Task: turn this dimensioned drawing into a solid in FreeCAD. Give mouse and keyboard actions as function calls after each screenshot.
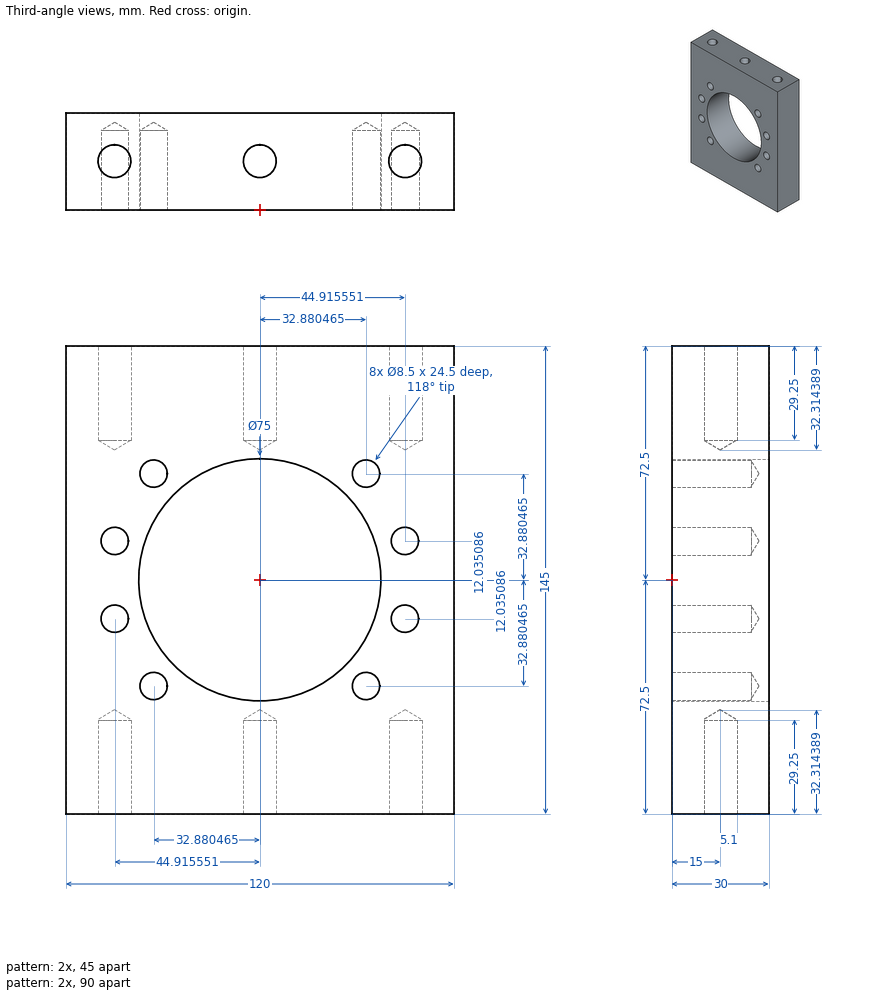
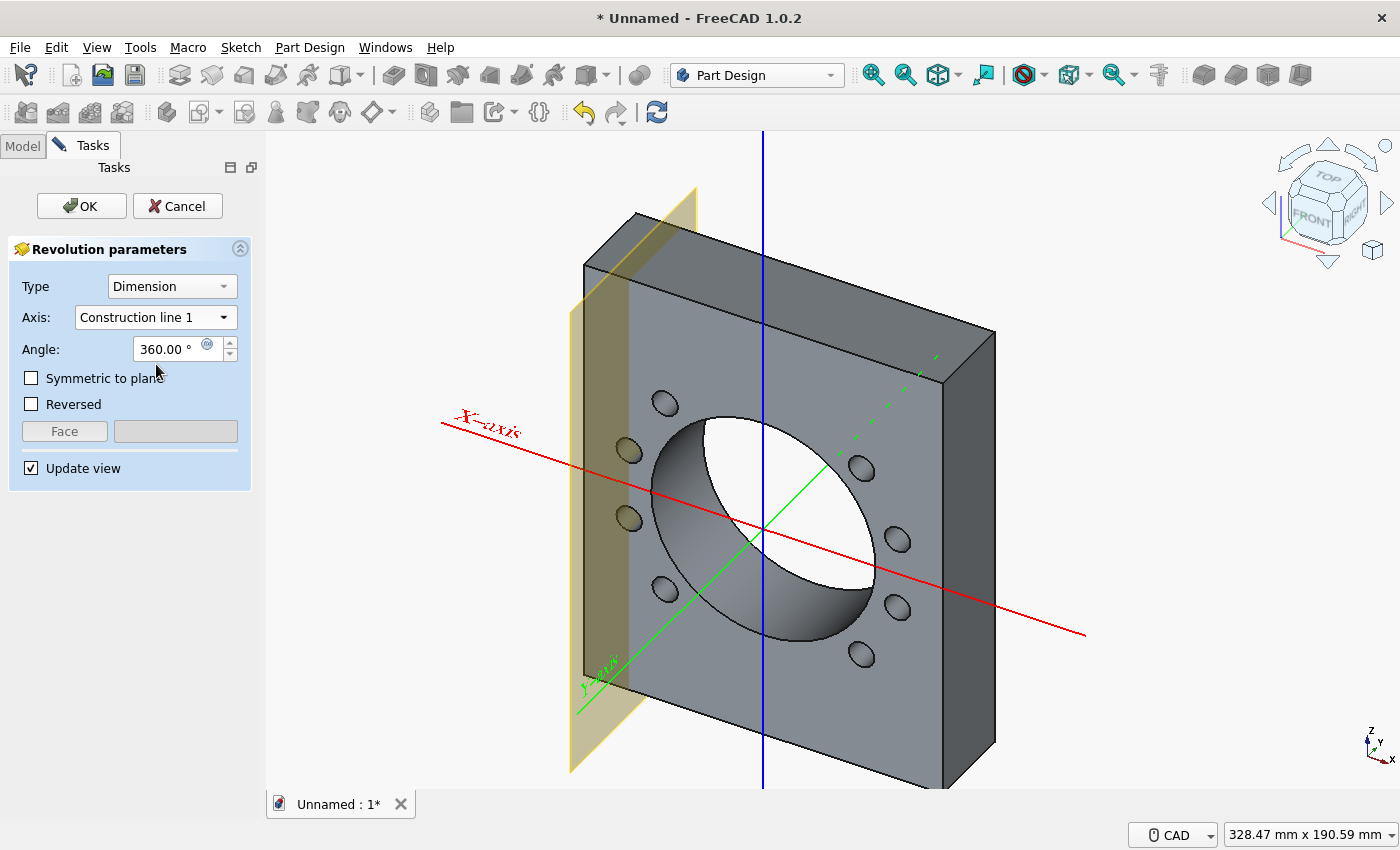
click(82, 206)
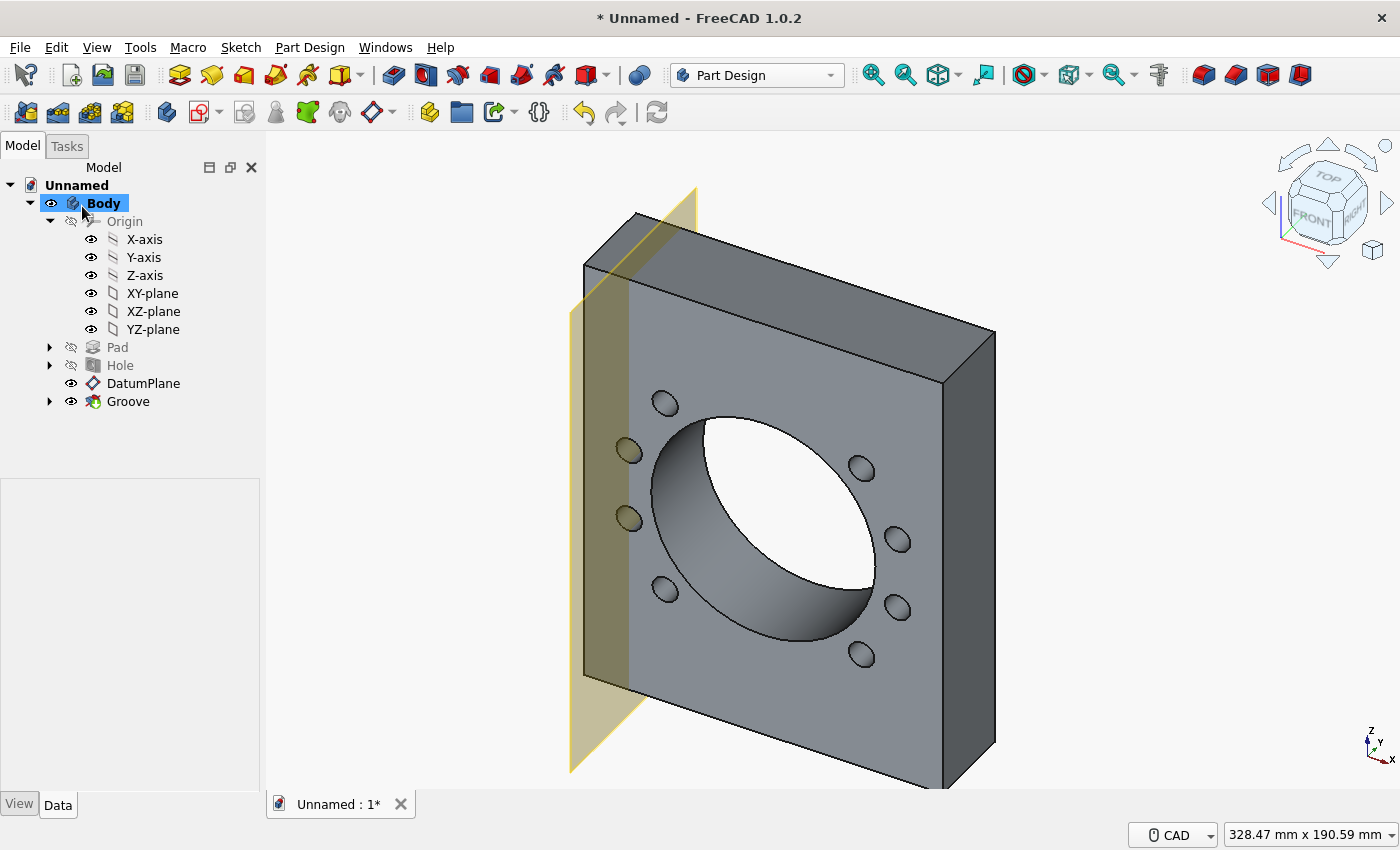
click(116, 383)
key(space)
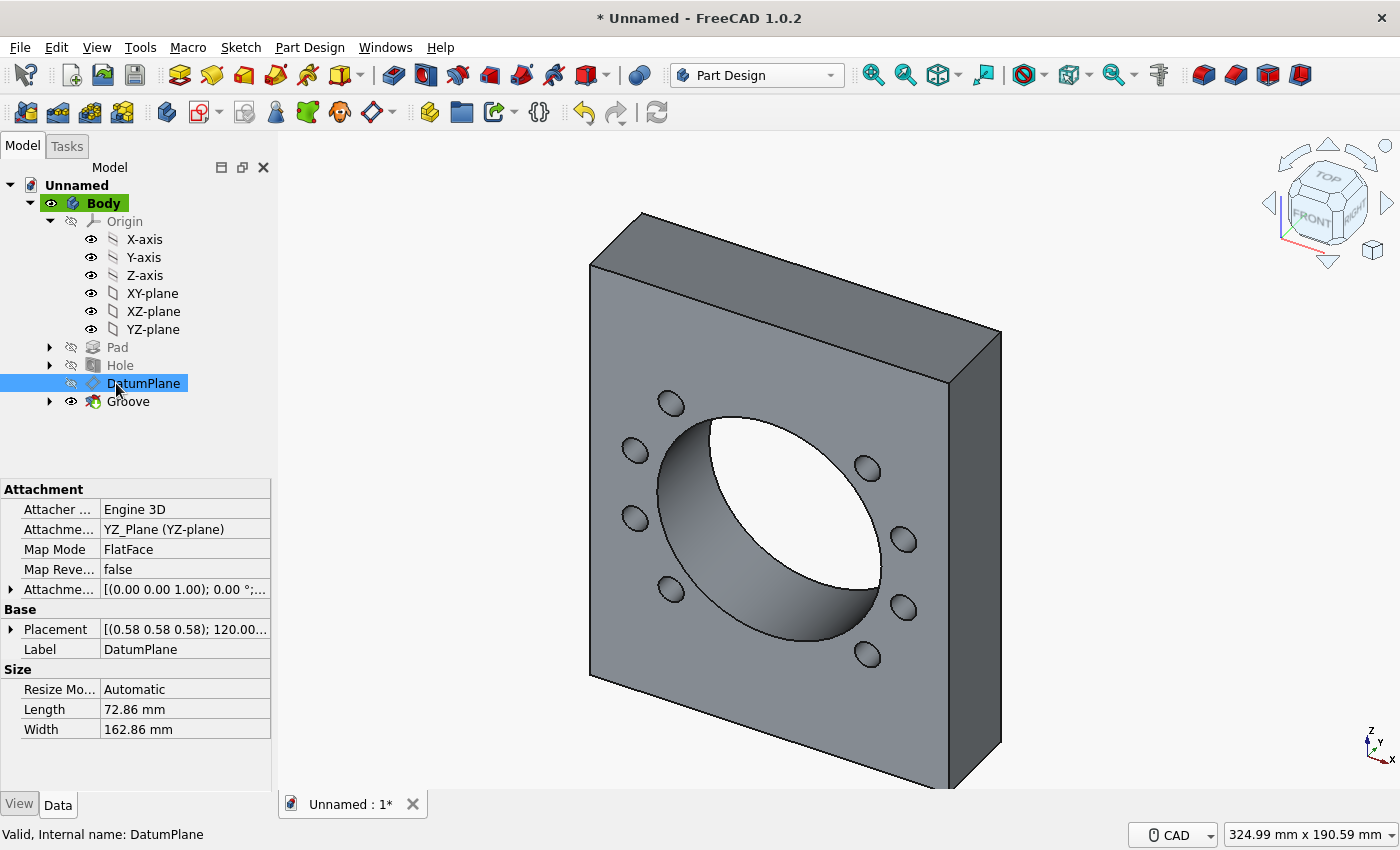
click(874, 76)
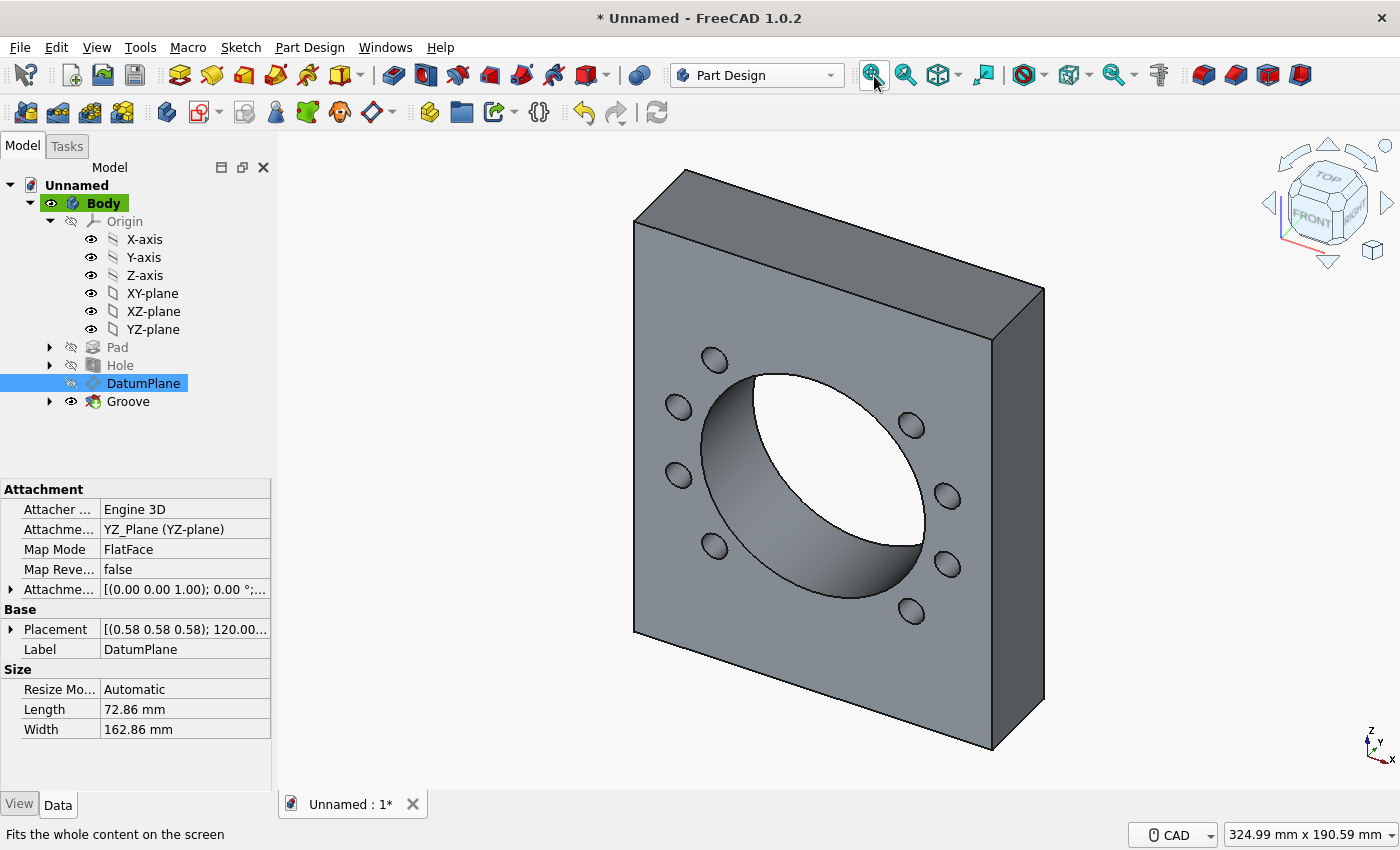
click(116, 401)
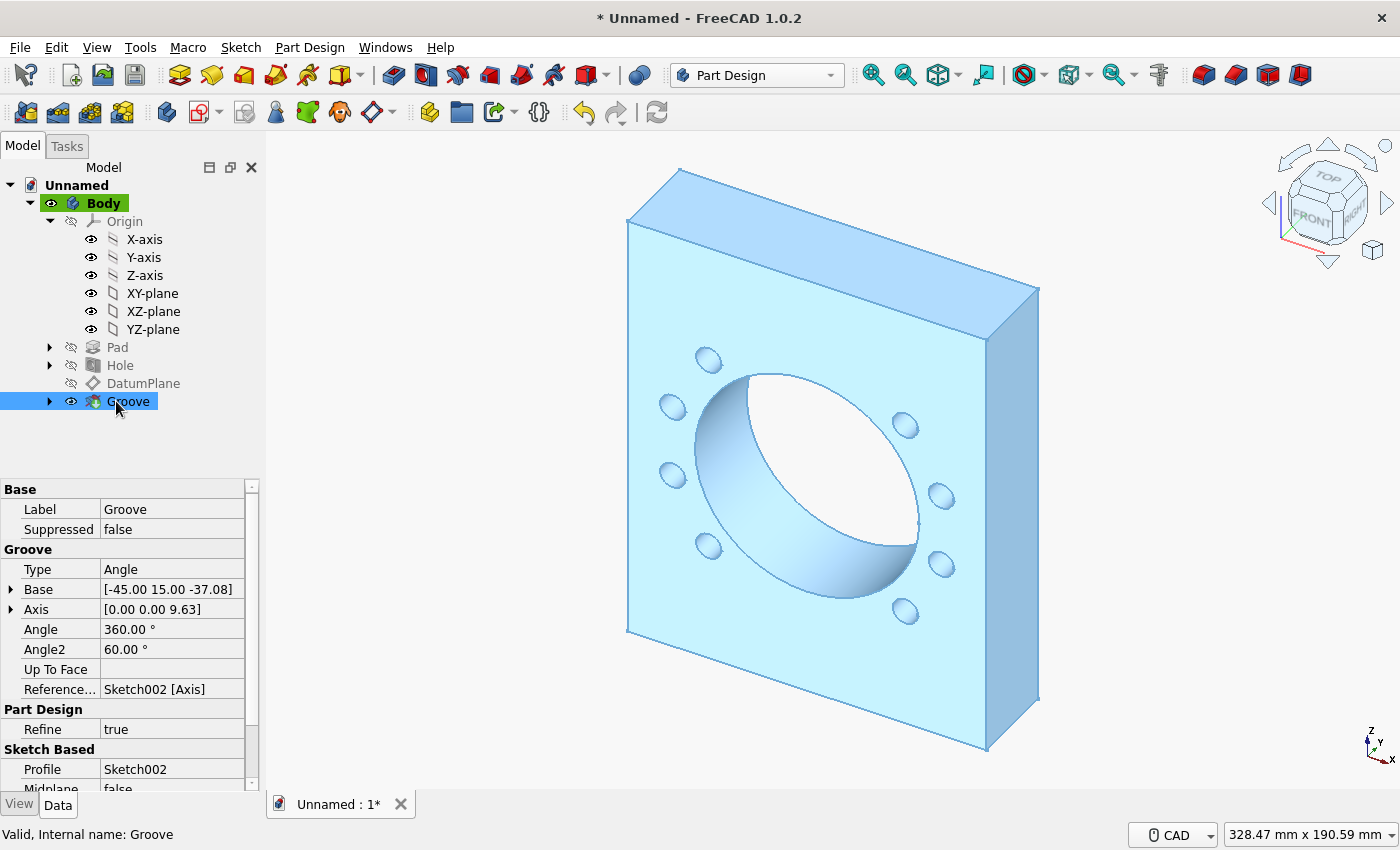
click(58, 112)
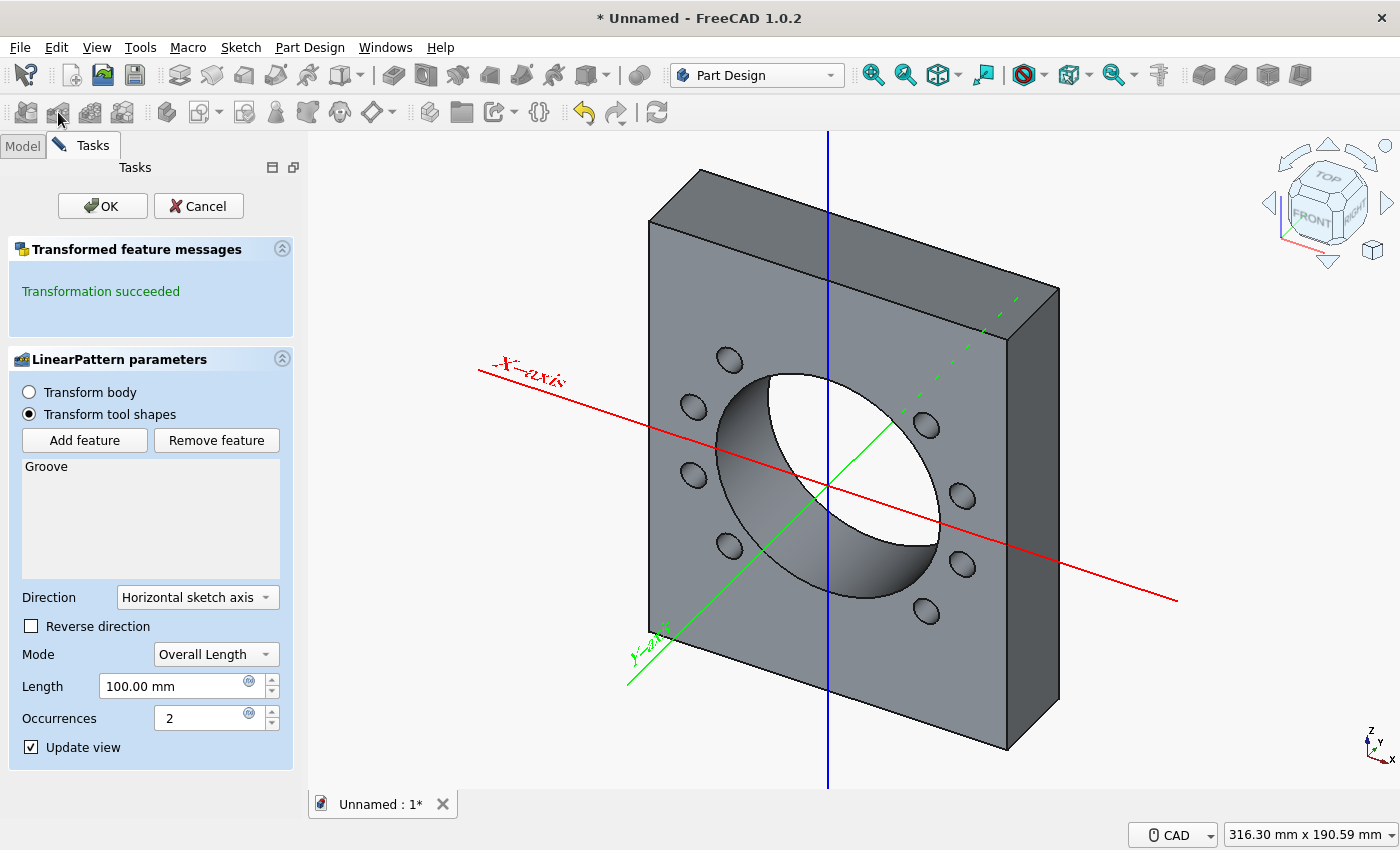
click(198, 598)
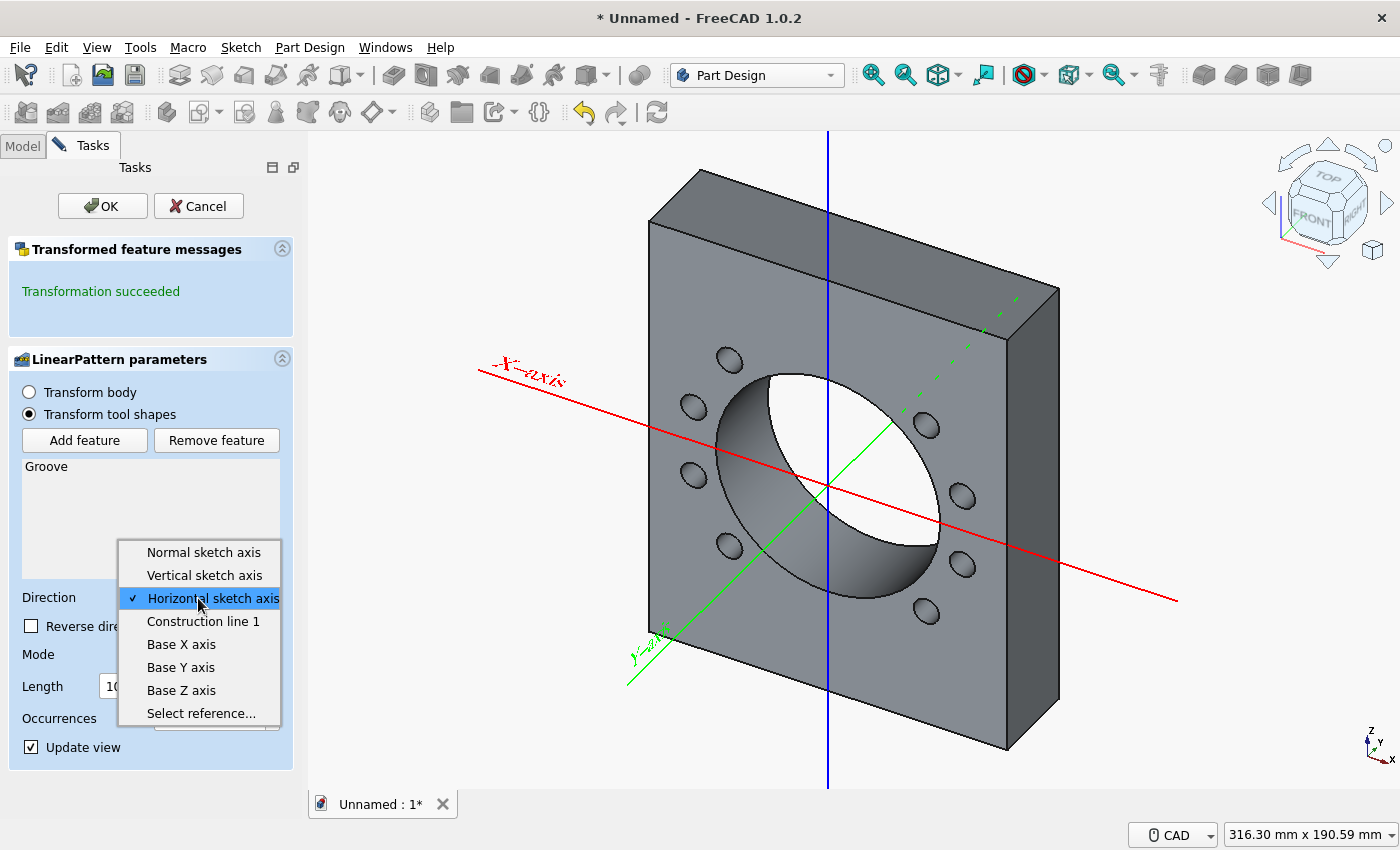
click(198, 644)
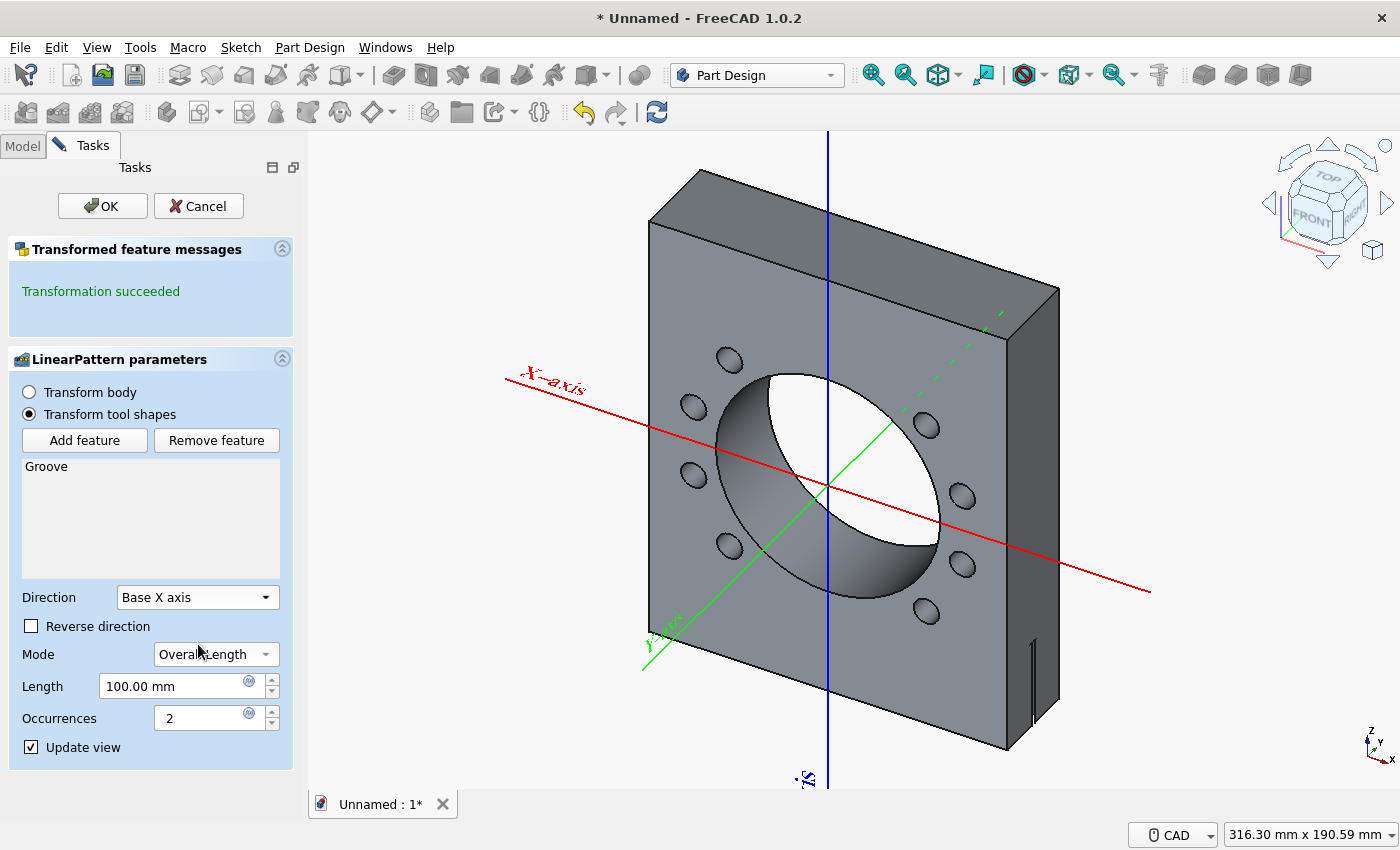
click(217, 654)